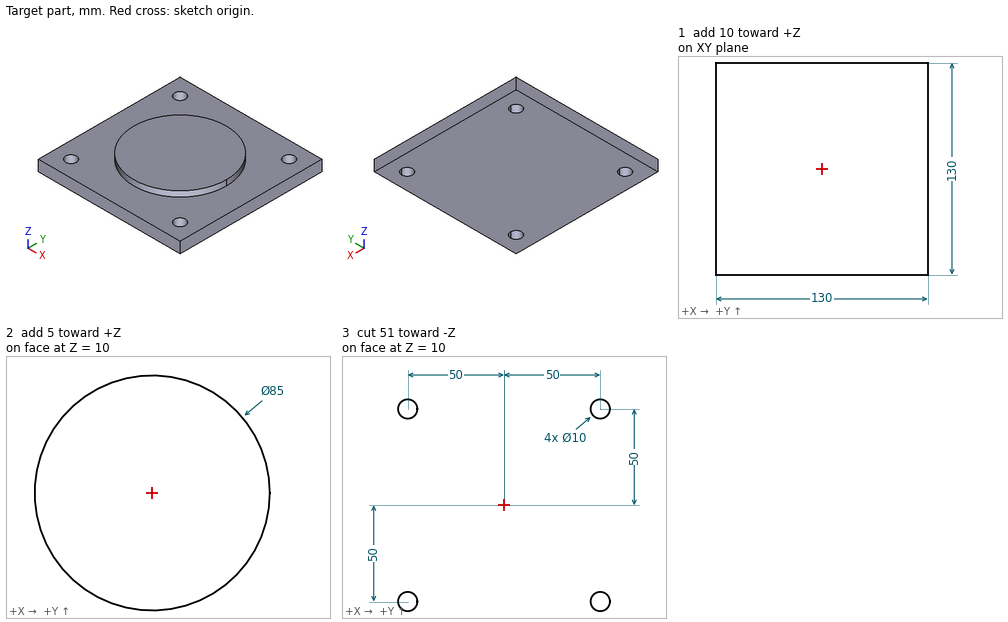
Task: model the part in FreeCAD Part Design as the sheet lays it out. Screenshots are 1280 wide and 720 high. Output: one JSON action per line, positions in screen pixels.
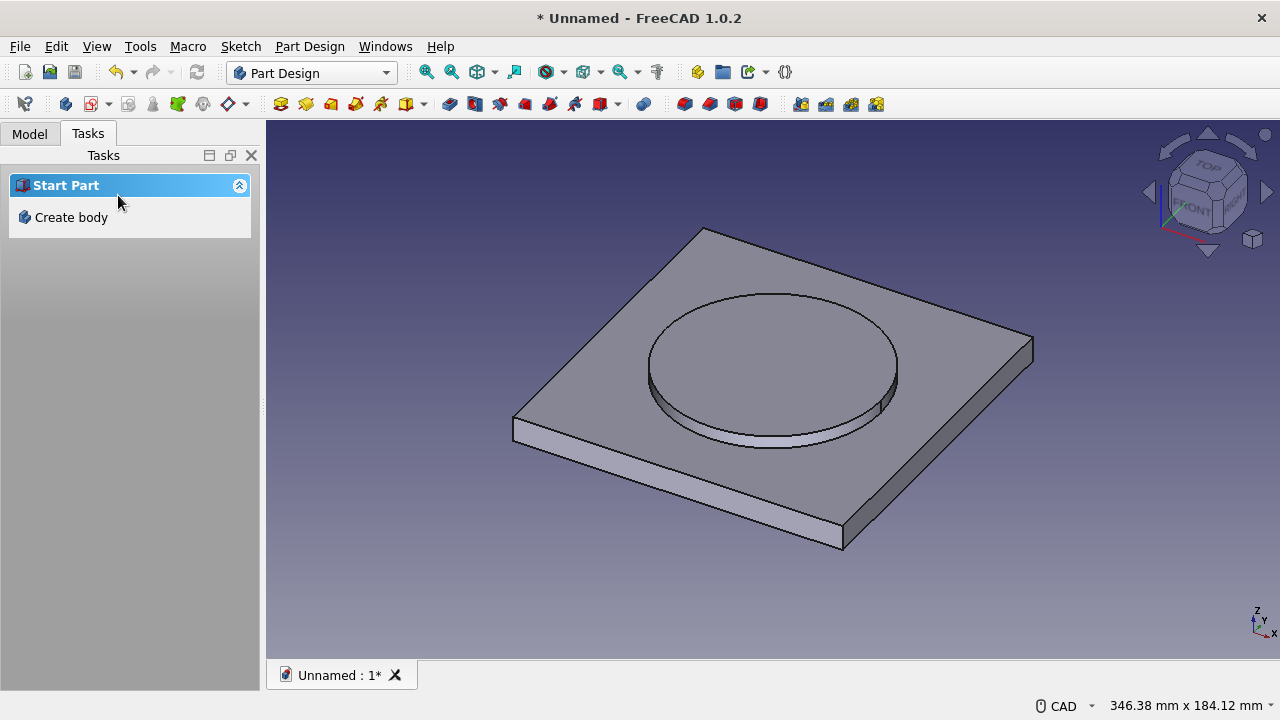
{"action": "left_click", "coordinate": [922, 353]}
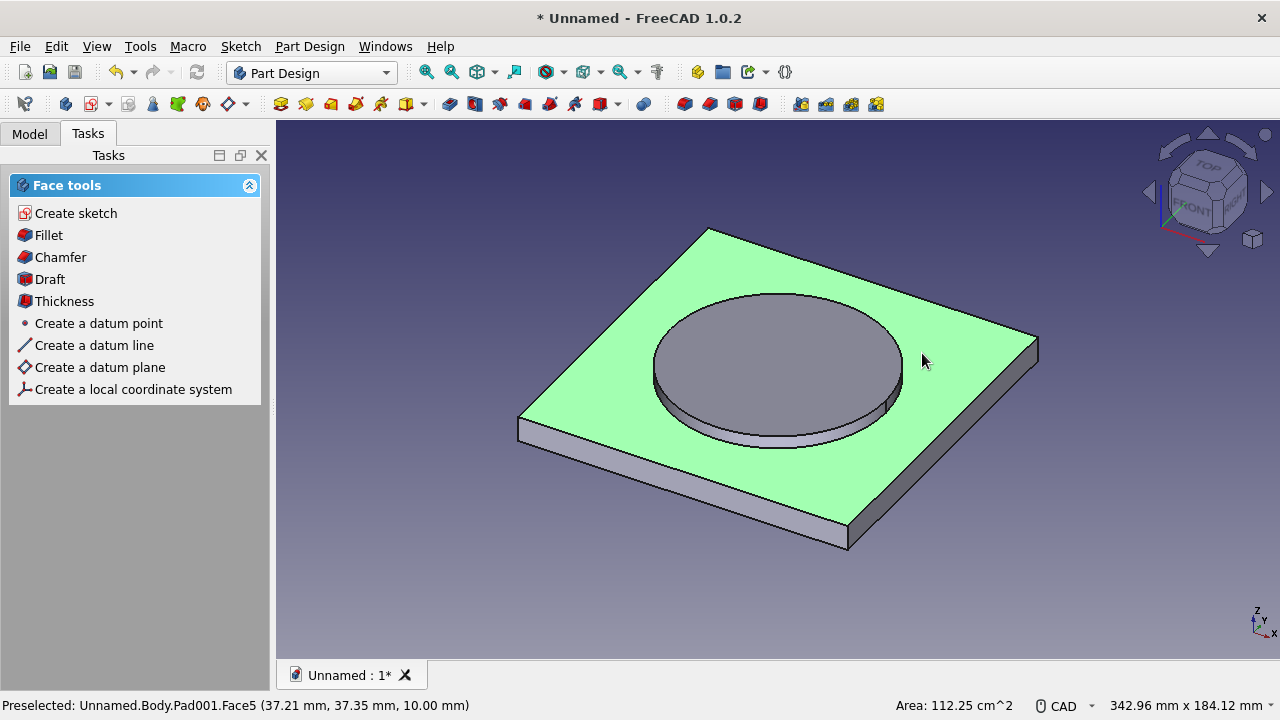
{"action": "left_click", "coordinate": [90, 104]}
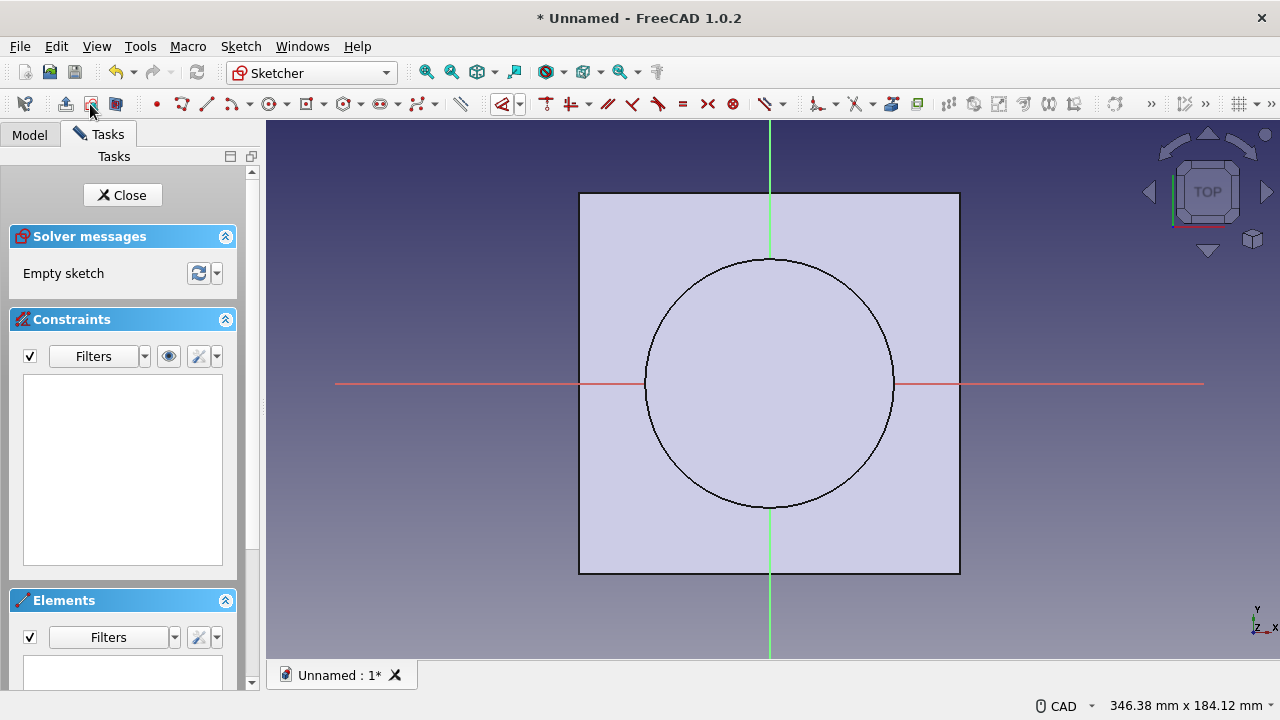
{"action": "left_click", "coordinate": [116, 104]}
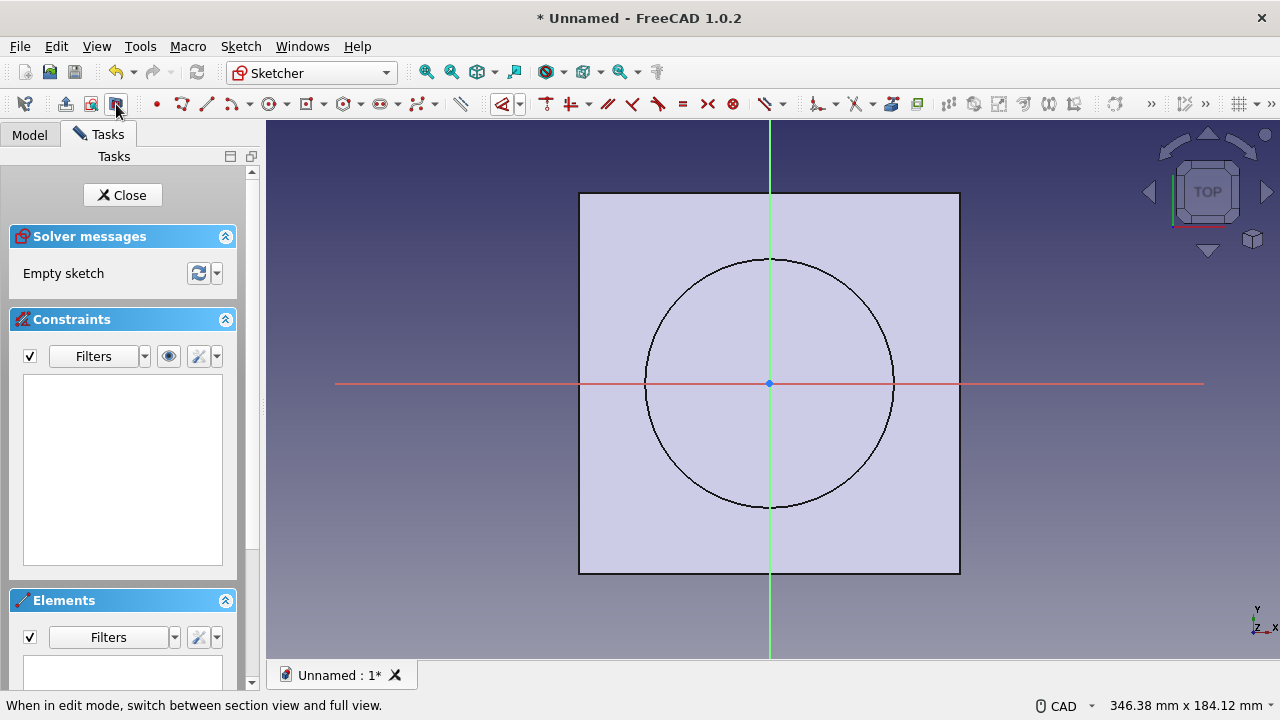
{"action": "left_click", "coordinate": [268, 104]}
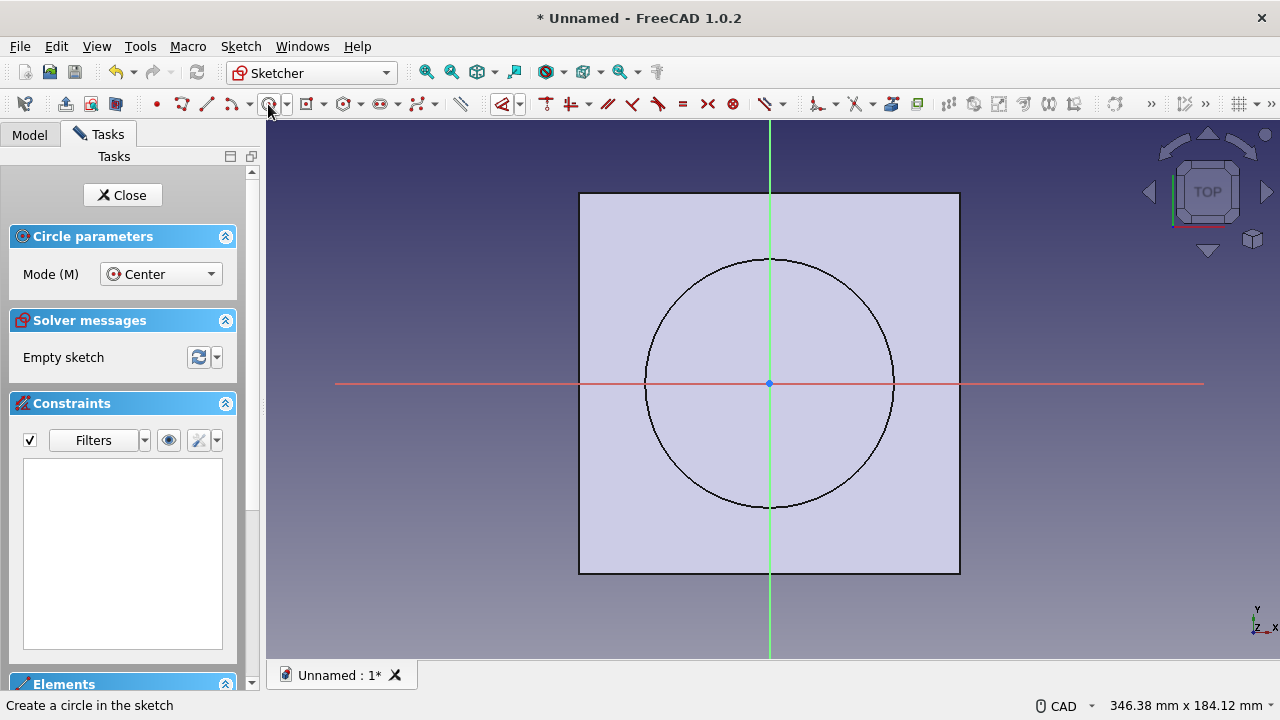
{"action": "scroll", "coordinate": [916, 237], "scroll_direction": "up", "scroll_amount": 3}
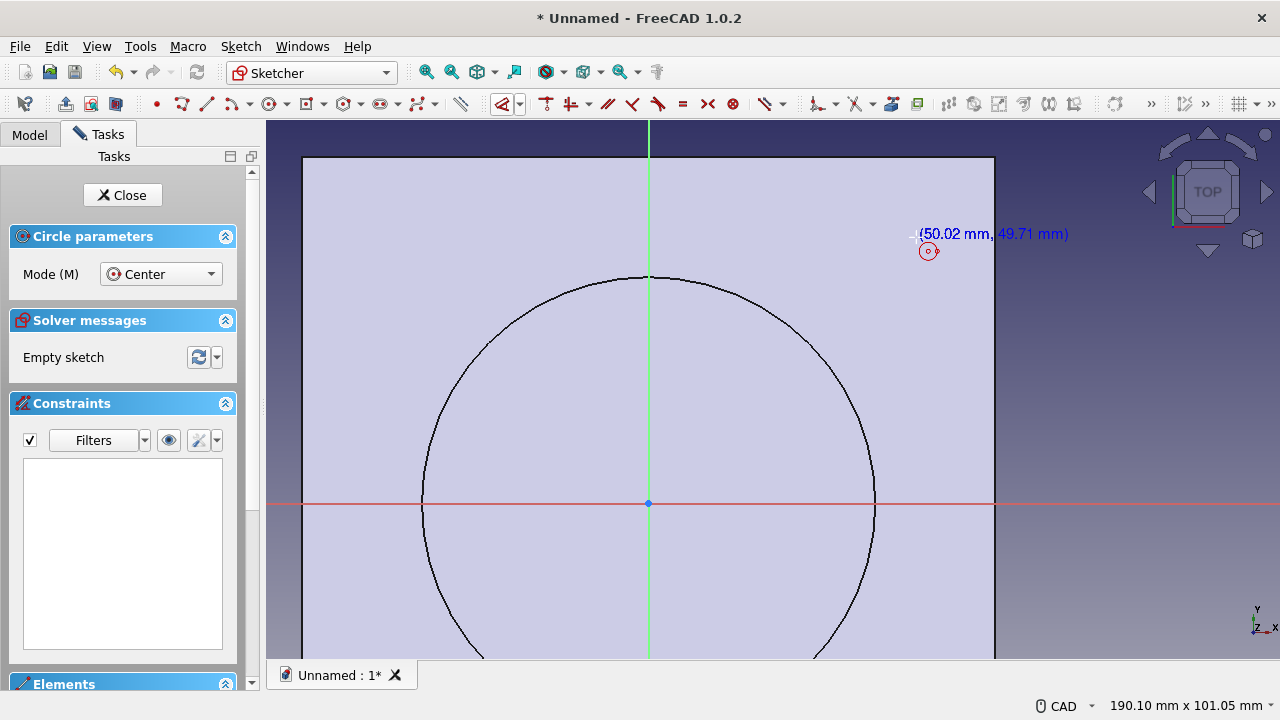
{"action": "left_click", "coordinate": [915, 237]}
{"action": "left_click", "coordinate": [934, 218]}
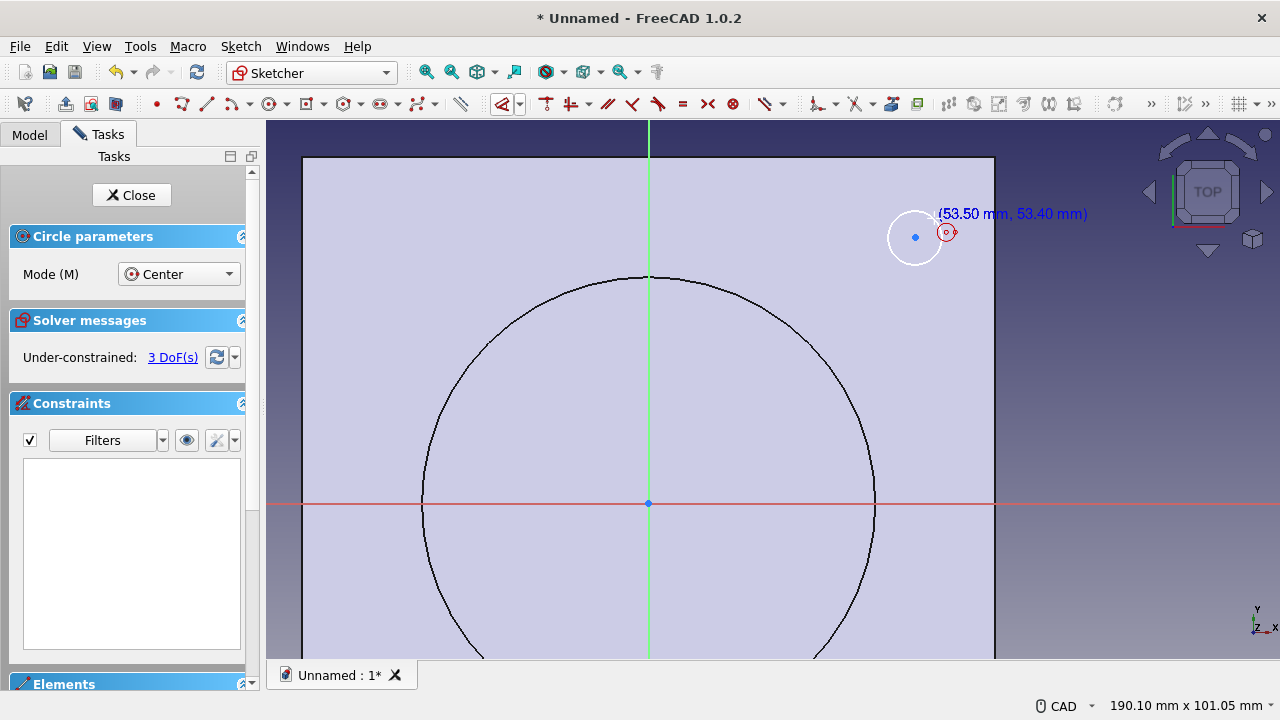
{"action": "left_click", "coordinate": [382, 237]}
{"action": "left_click", "coordinate": [401, 218]}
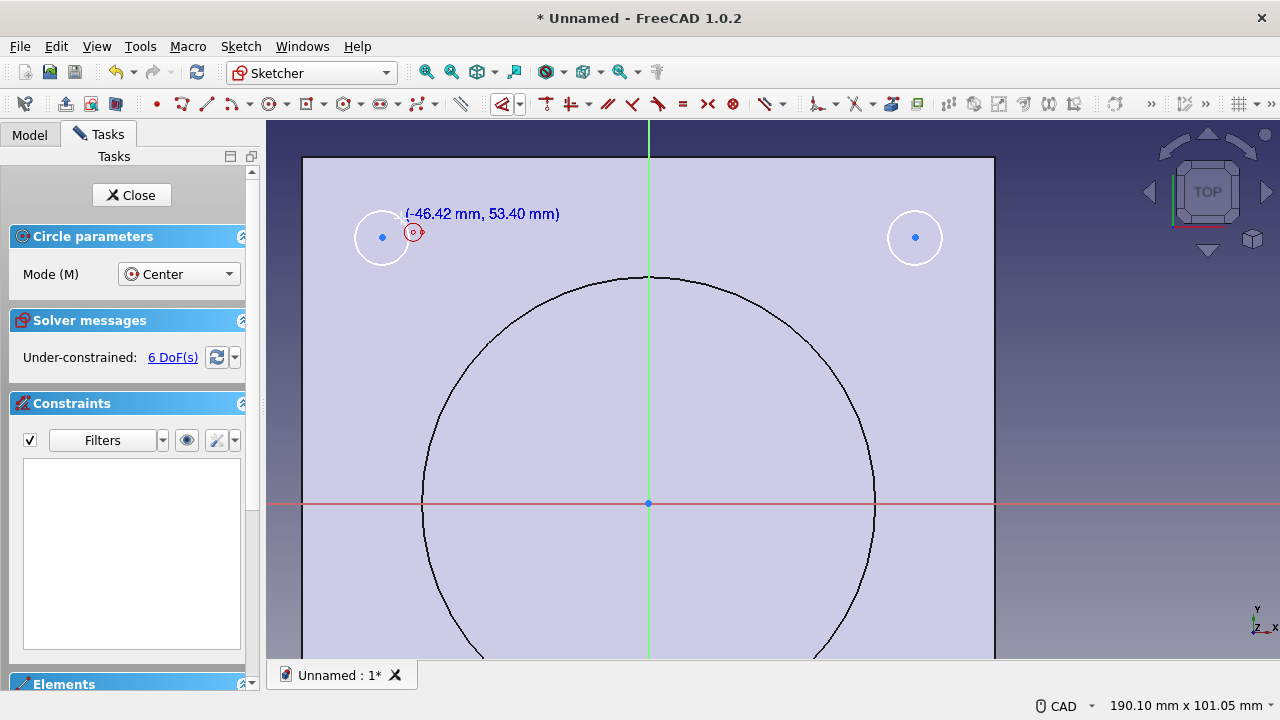
{"action": "scroll", "coordinate": [772, 250], "scroll_direction": "down", "scroll_amount": 3}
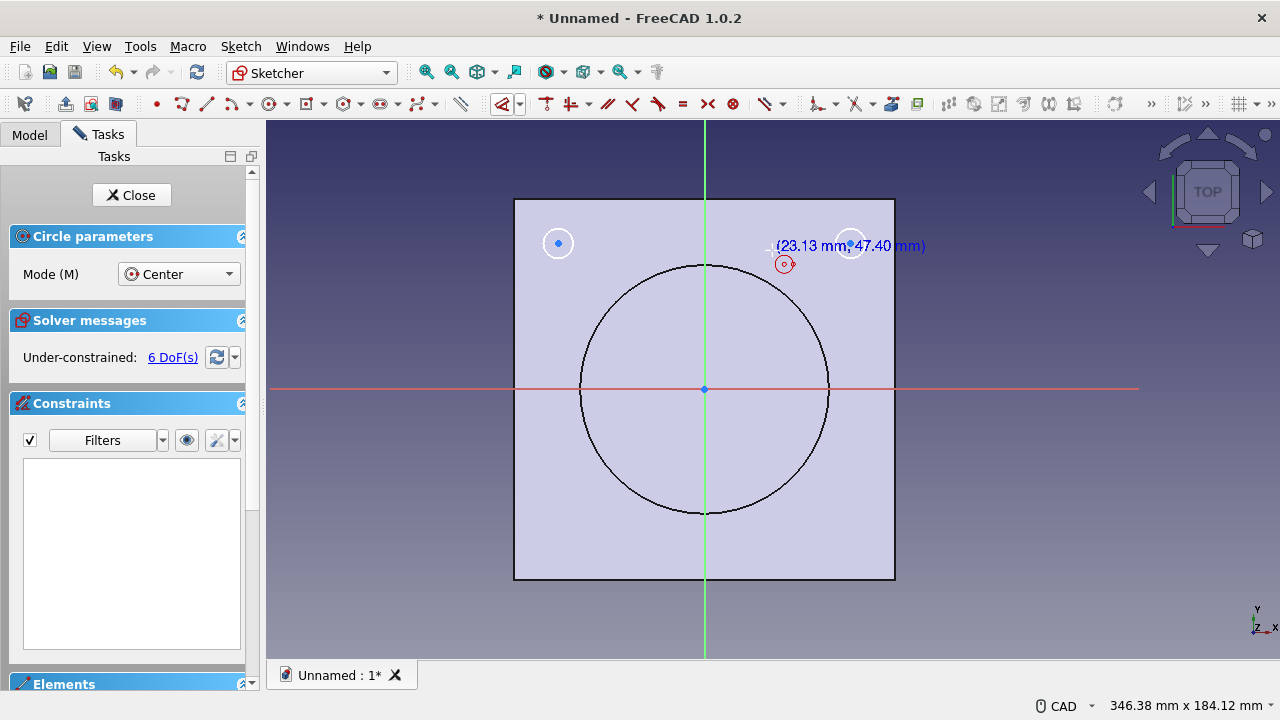
{"action": "scroll", "coordinate": [558, 536], "scroll_direction": "up", "scroll_amount": 3}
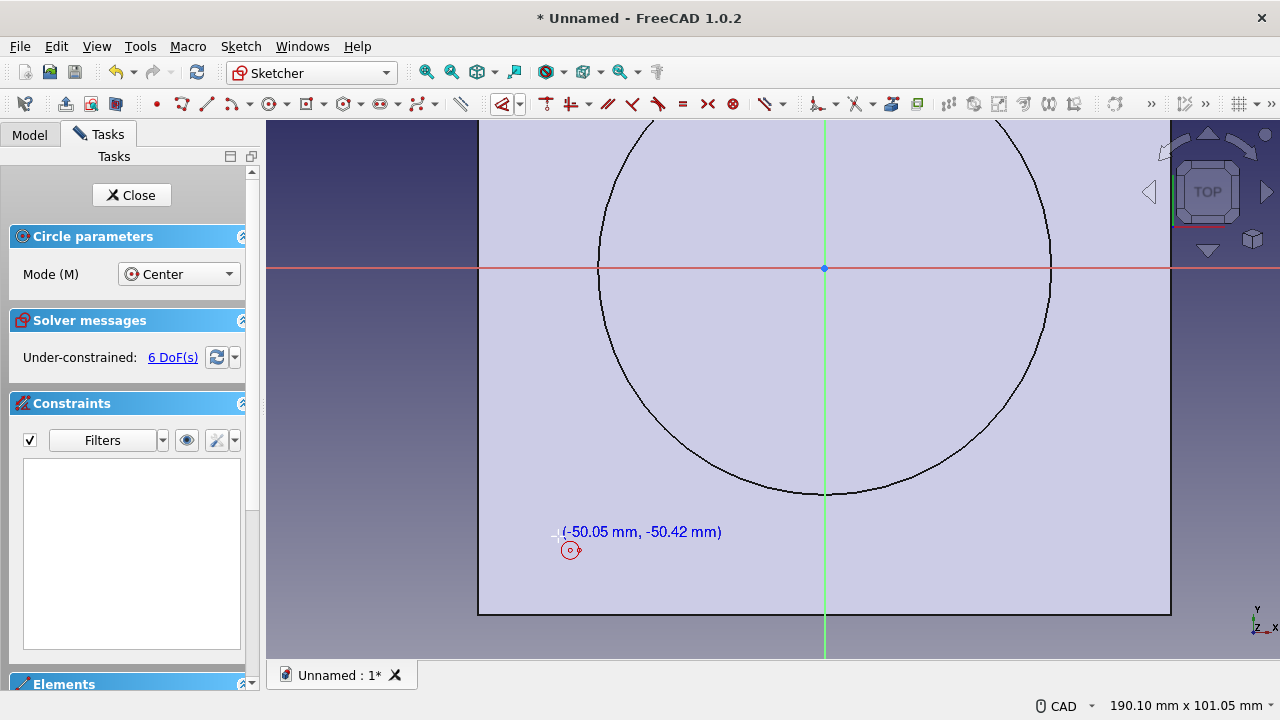
{"action": "left_click", "coordinate": [558, 535]}
{"action": "left_click", "coordinate": [577, 516]}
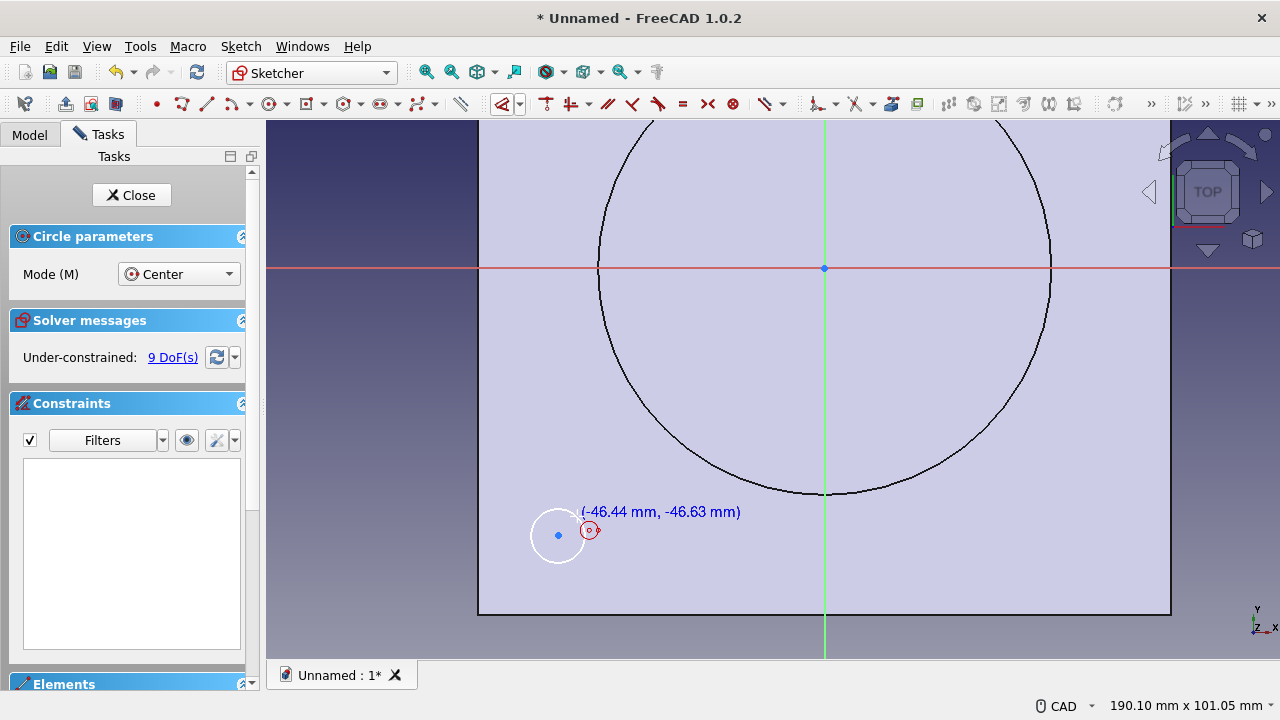
{"action": "left_click", "coordinate": [1091, 535]}
{"action": "left_click", "coordinate": [1110, 516]}
{"action": "key", "text": "Escape"}